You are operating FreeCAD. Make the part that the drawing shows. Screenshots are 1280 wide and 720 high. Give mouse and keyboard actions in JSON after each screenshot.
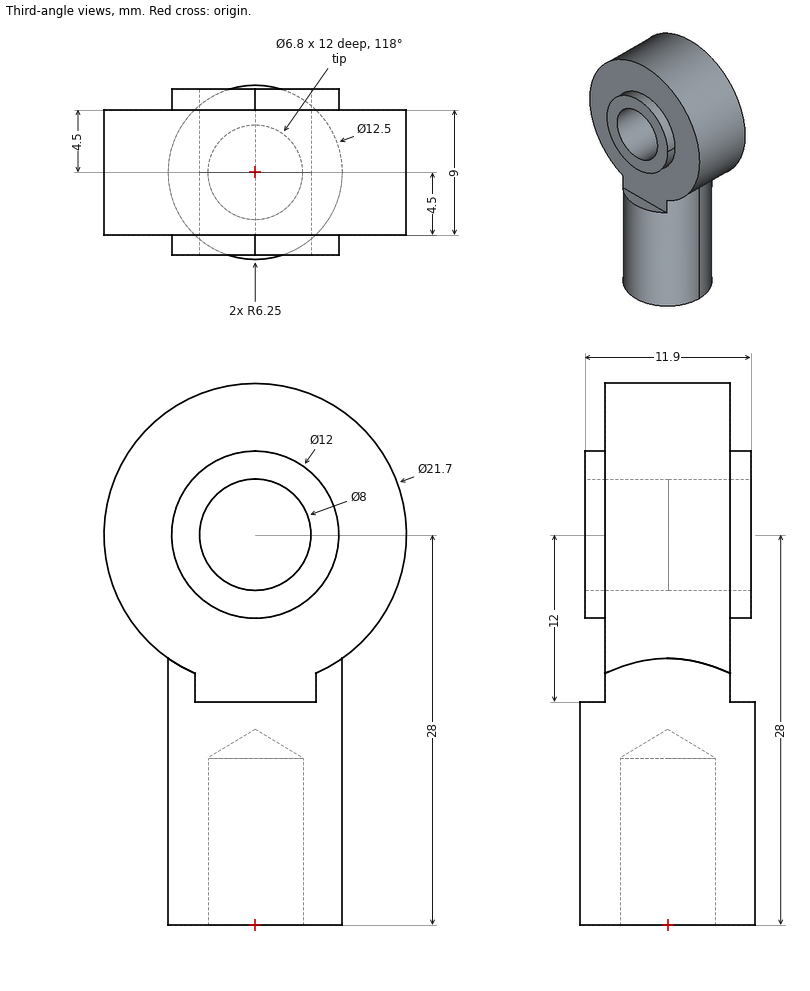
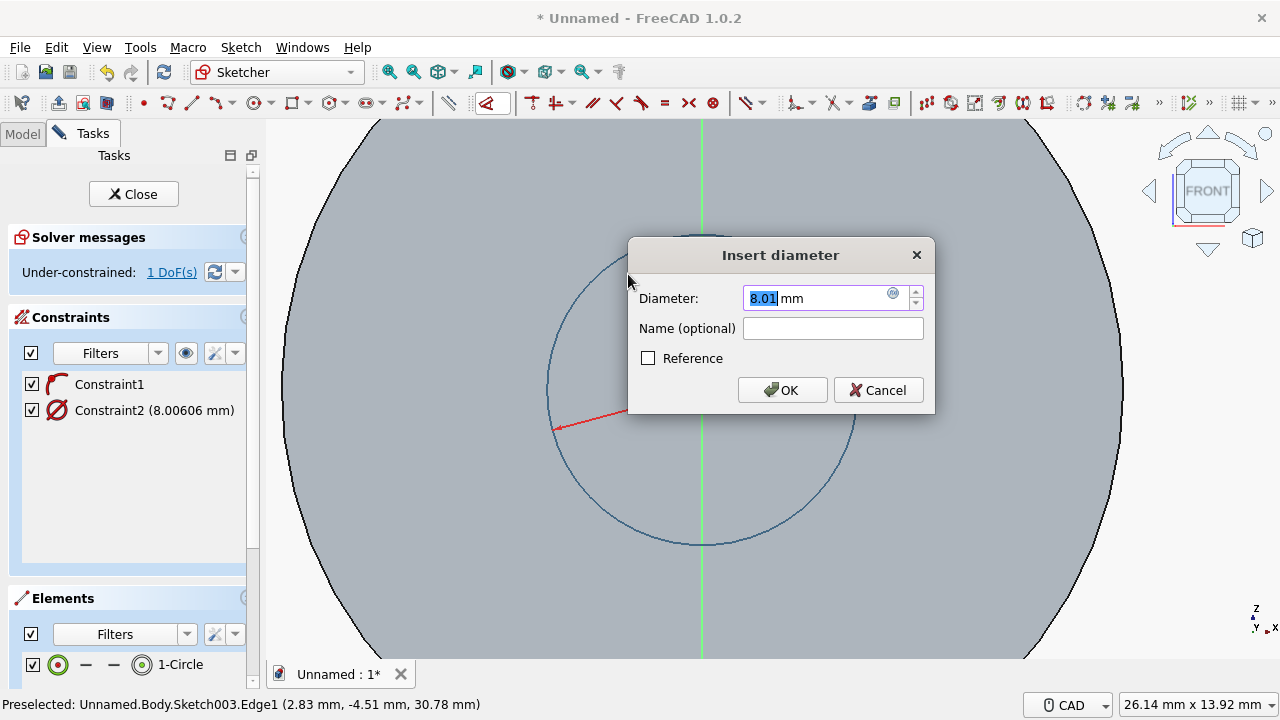
{"action": "type", "text": "8"}
{"action": "key", "text": "Return"}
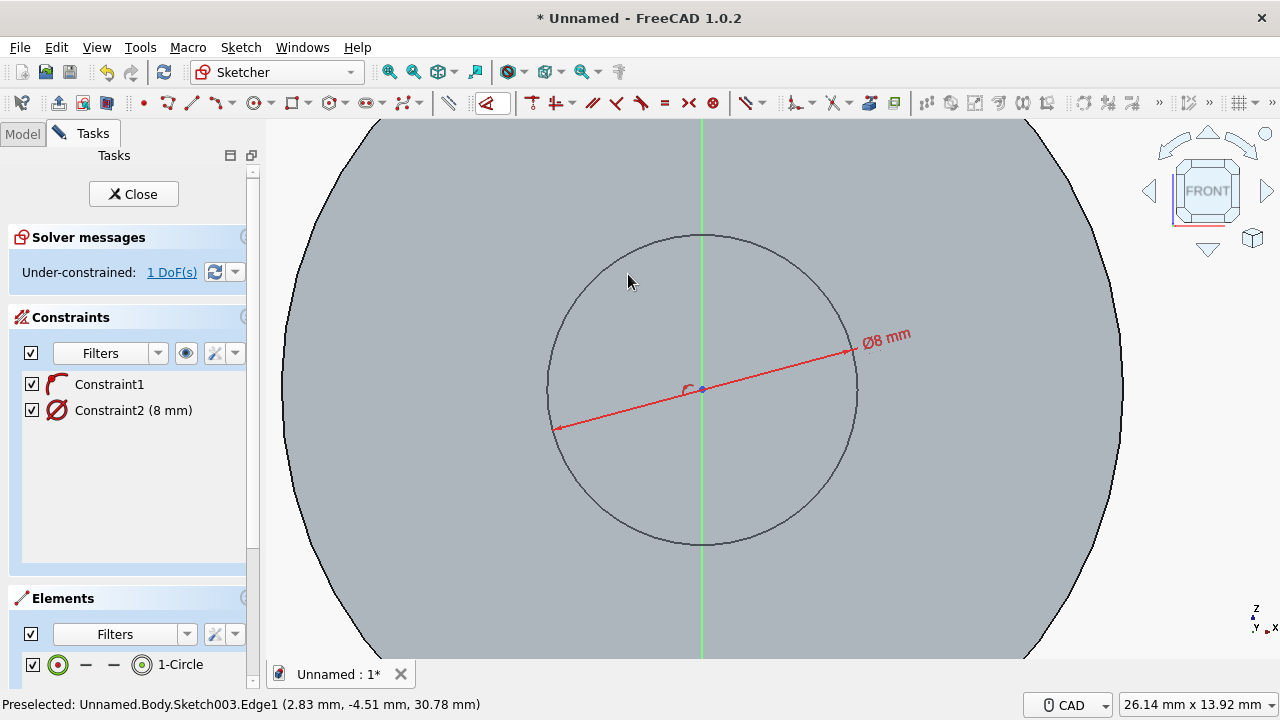
{"action": "left_click", "coordinate": [702, 390]}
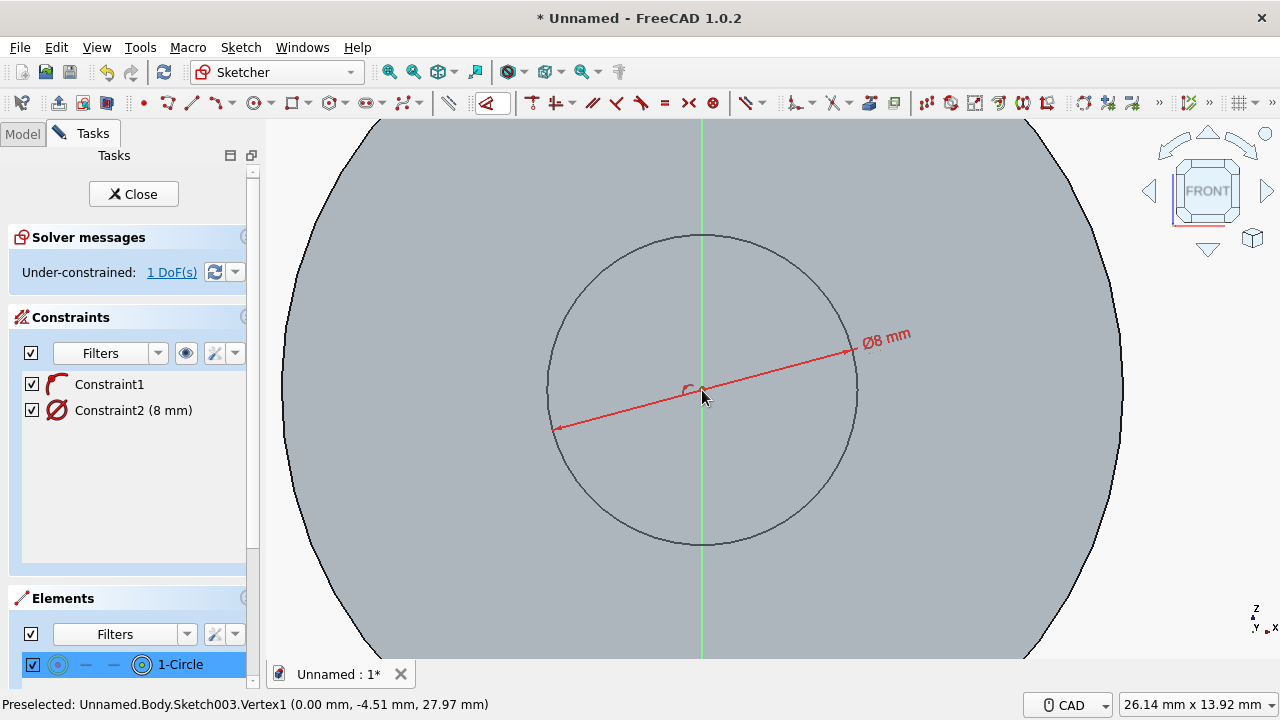
{"action": "key", "text": "i"}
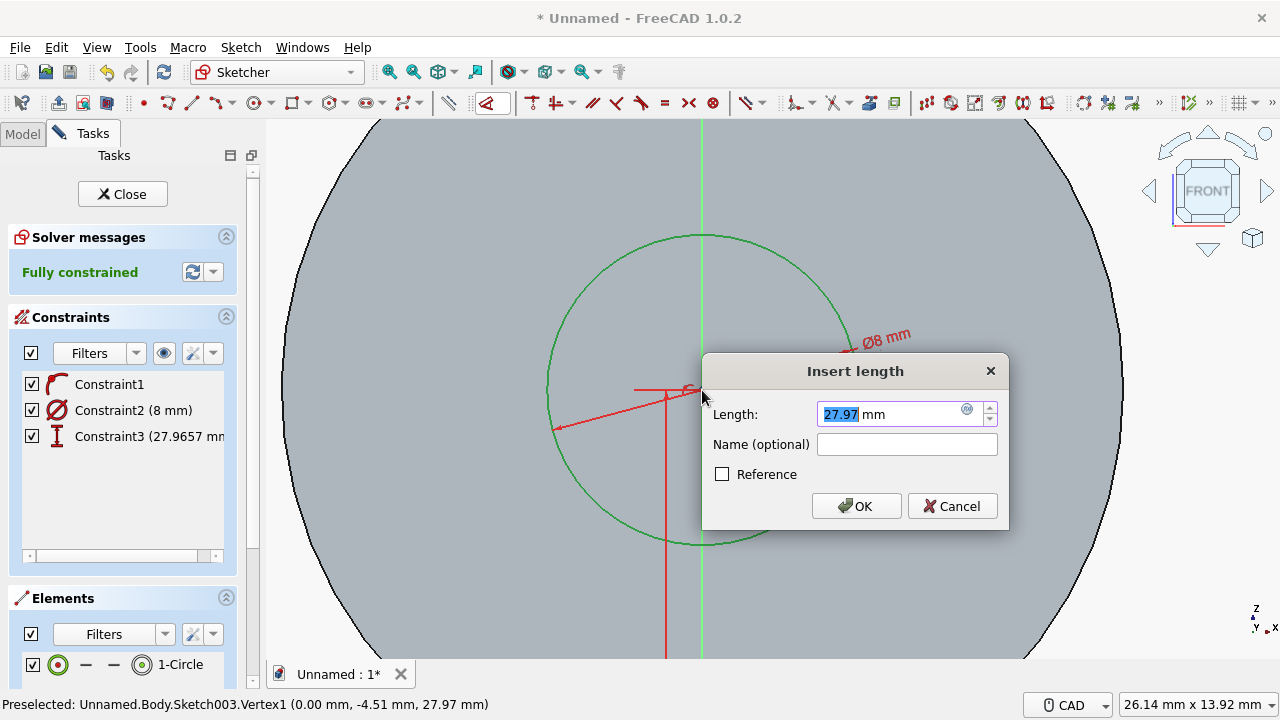
{"action": "type", "text": "28"}
{"action": "key", "text": "Return"}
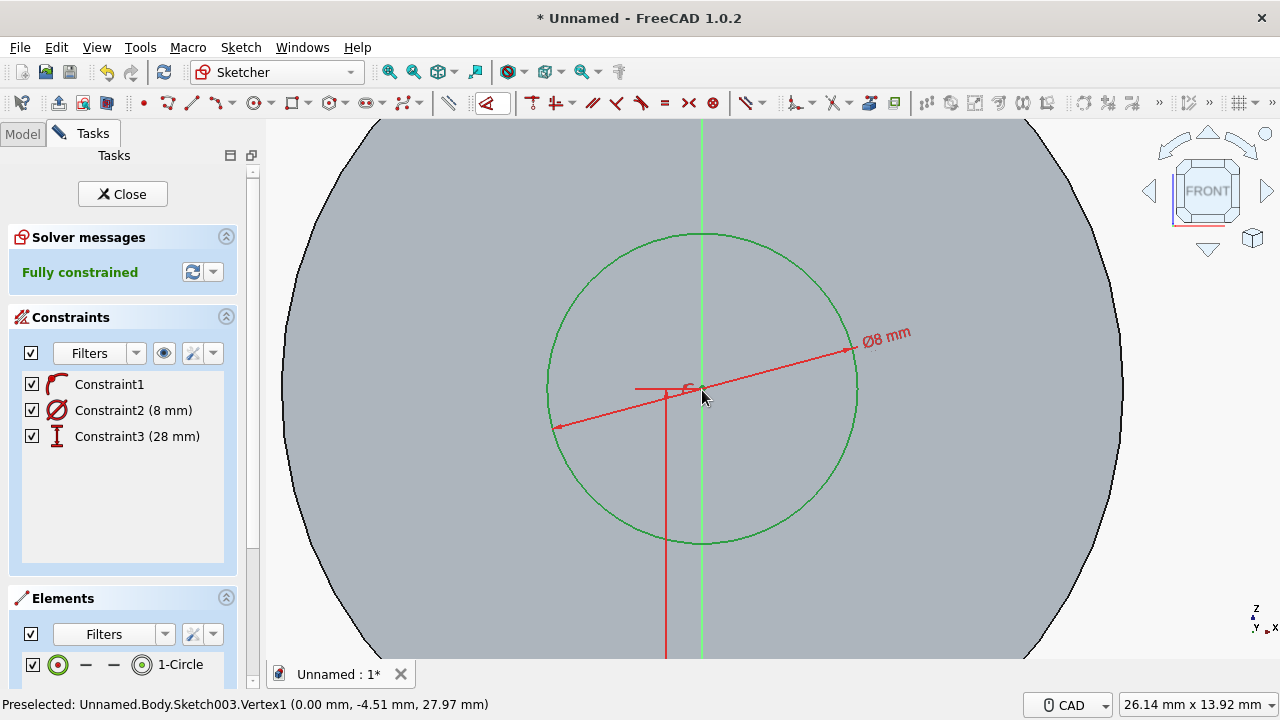
{"action": "left_click", "coordinate": [123, 194]}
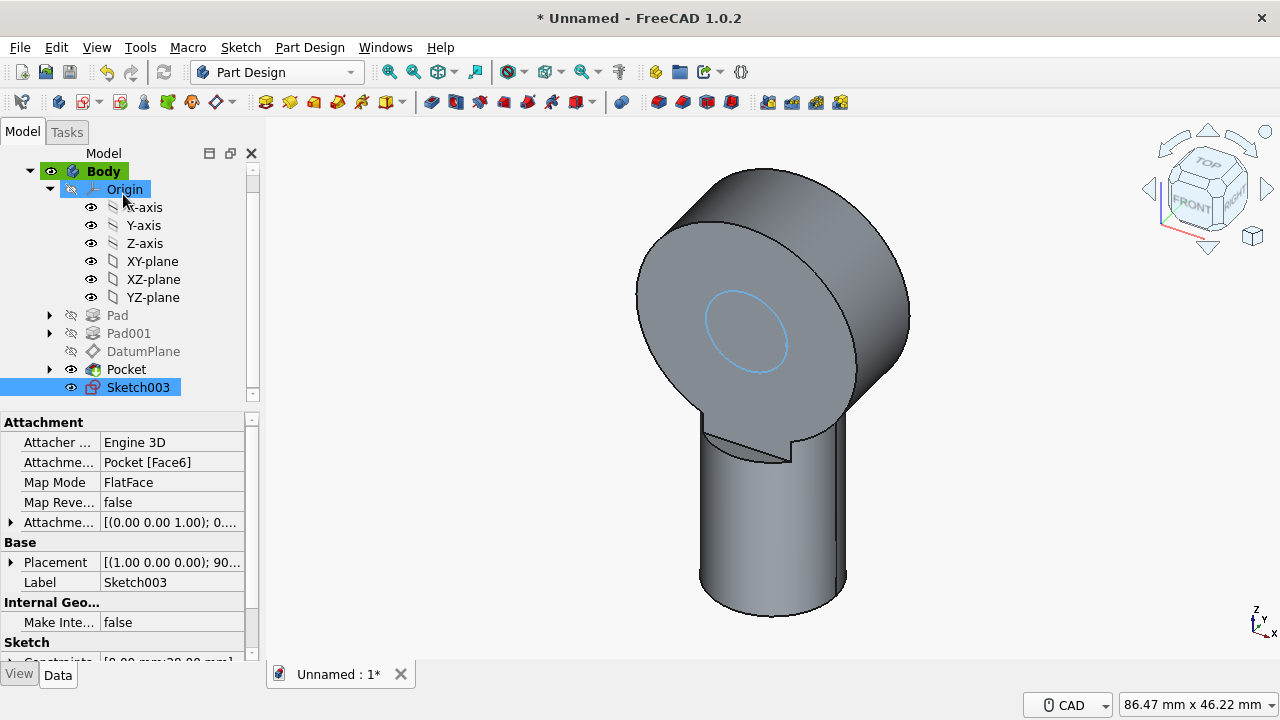
{"action": "left_click", "coordinate": [432, 102]}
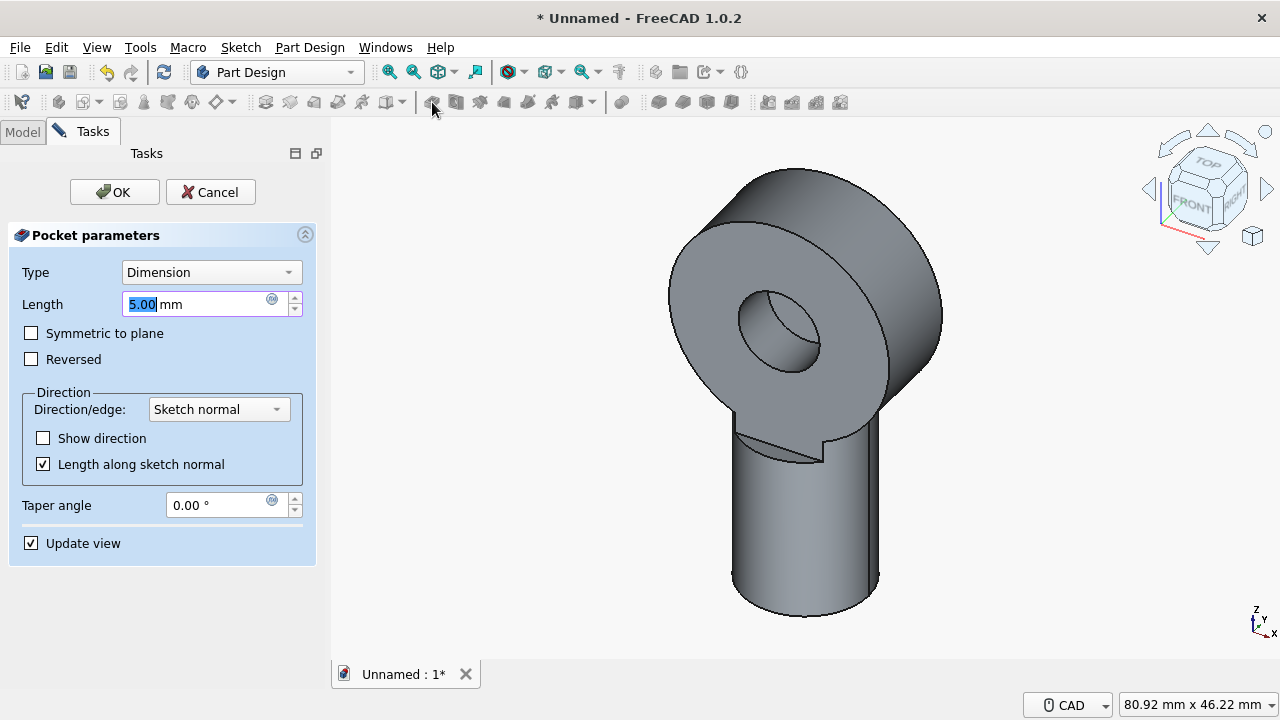
{"action": "left_click", "coordinate": [212, 272]}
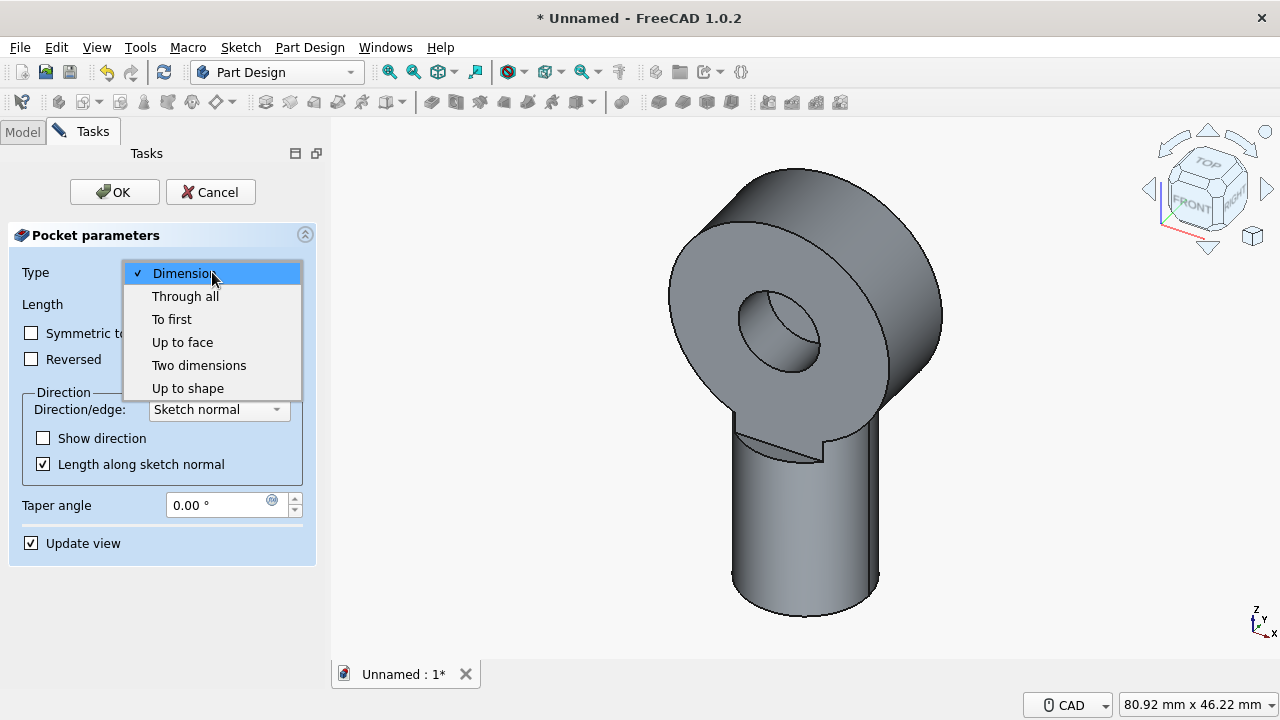
{"action": "left_click", "coordinate": [212, 296]}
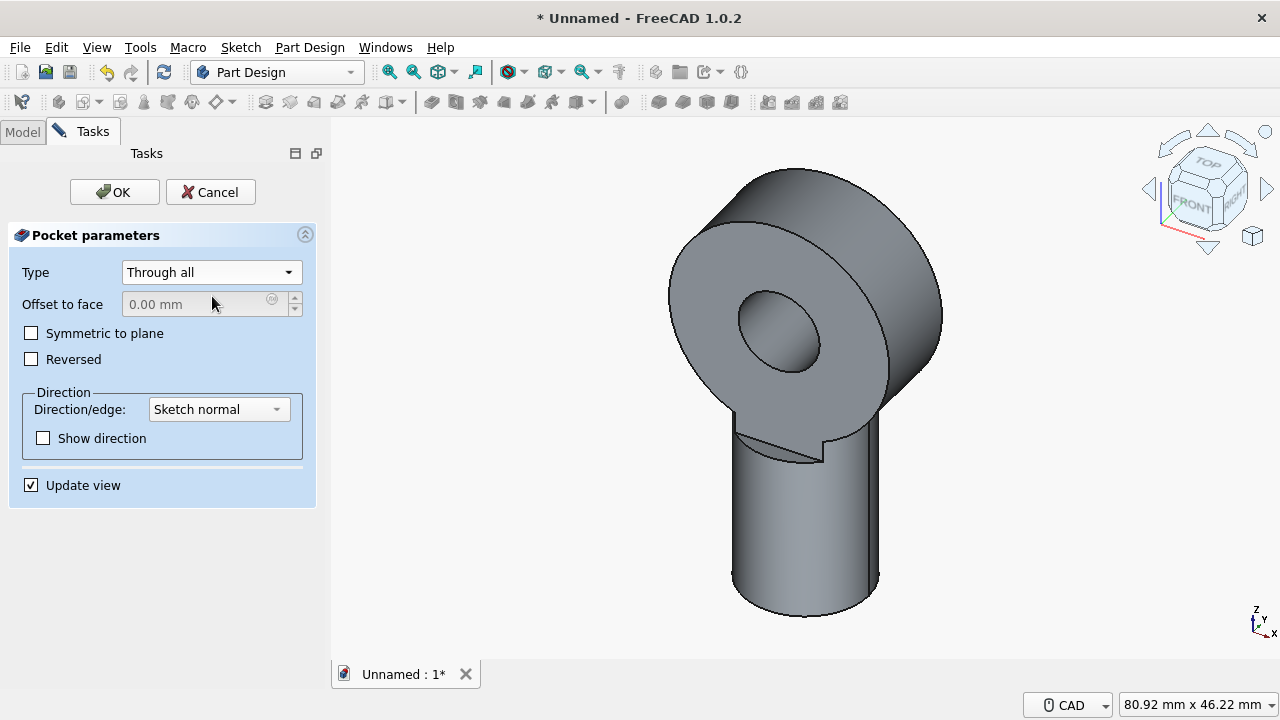
{"action": "left_click", "coordinate": [115, 192]}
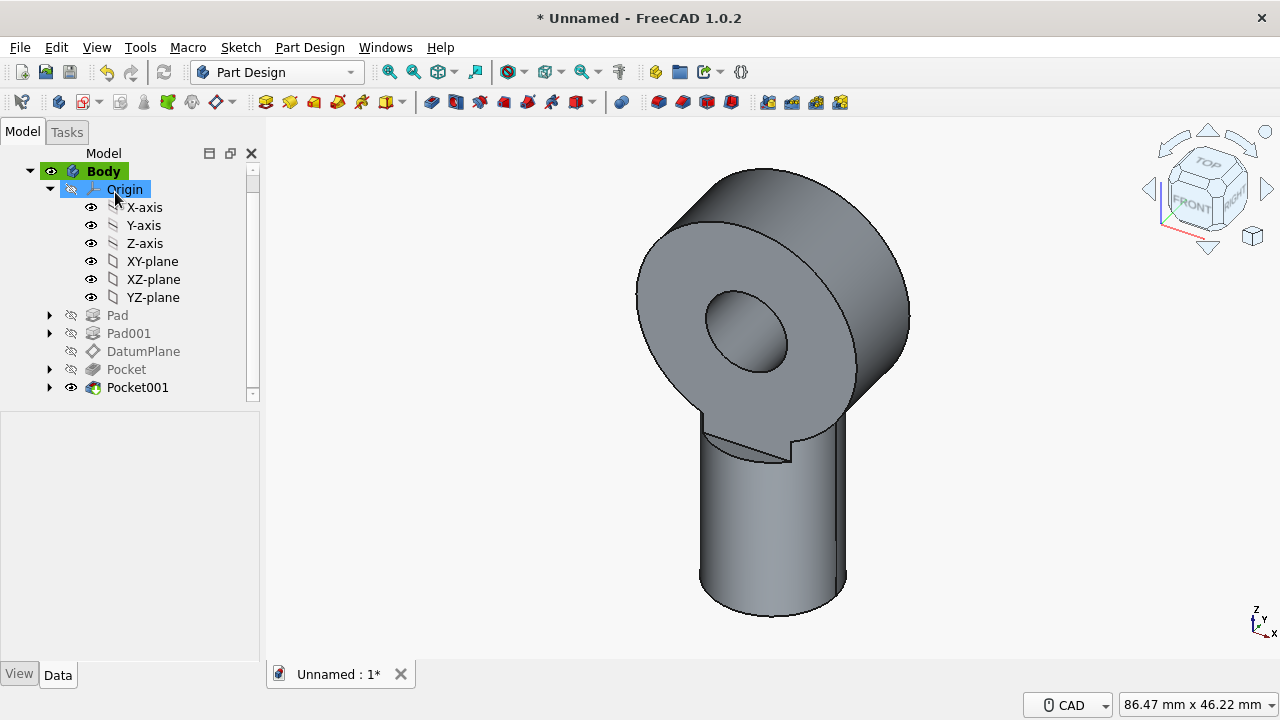
{"action": "left_click", "coordinate": [84, 102]}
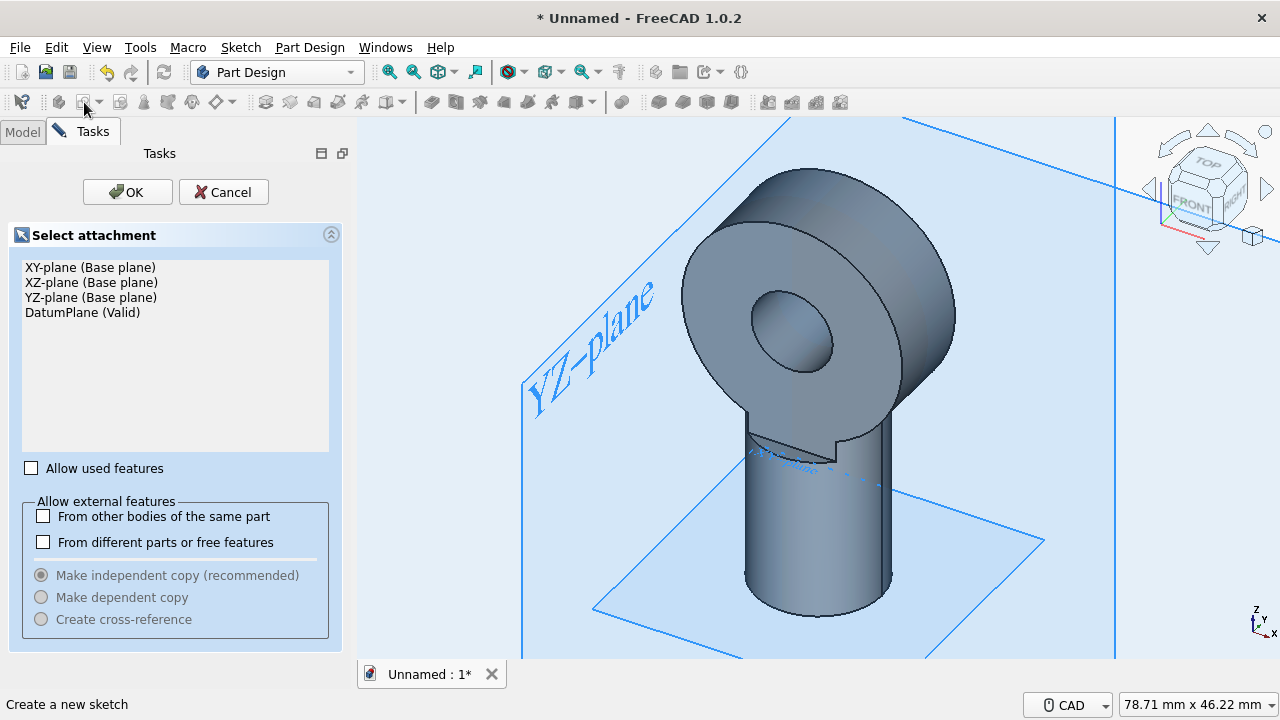
{"action": "left_click", "coordinate": [82, 268]}